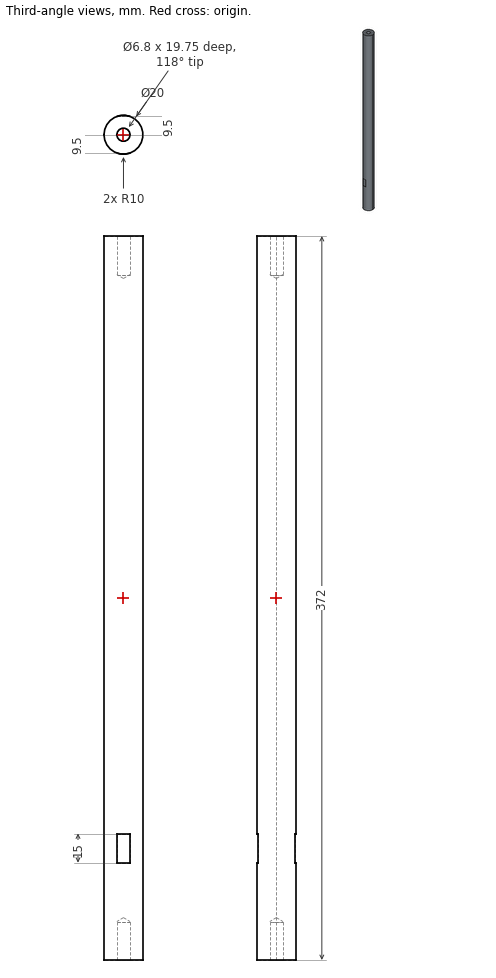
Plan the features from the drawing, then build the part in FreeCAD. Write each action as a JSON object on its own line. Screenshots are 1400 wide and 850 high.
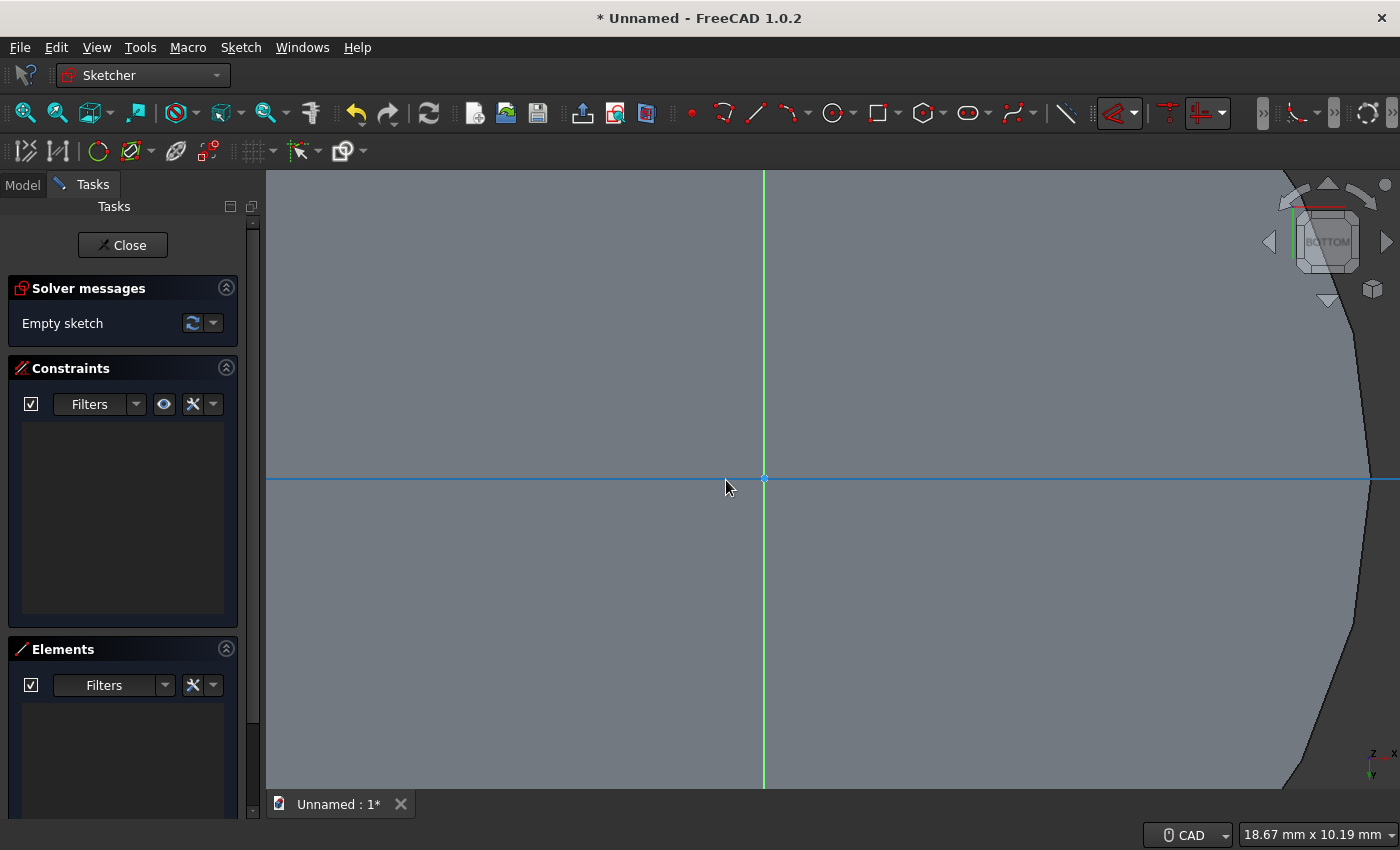
{"action": "left_click", "coordinate": [834, 114]}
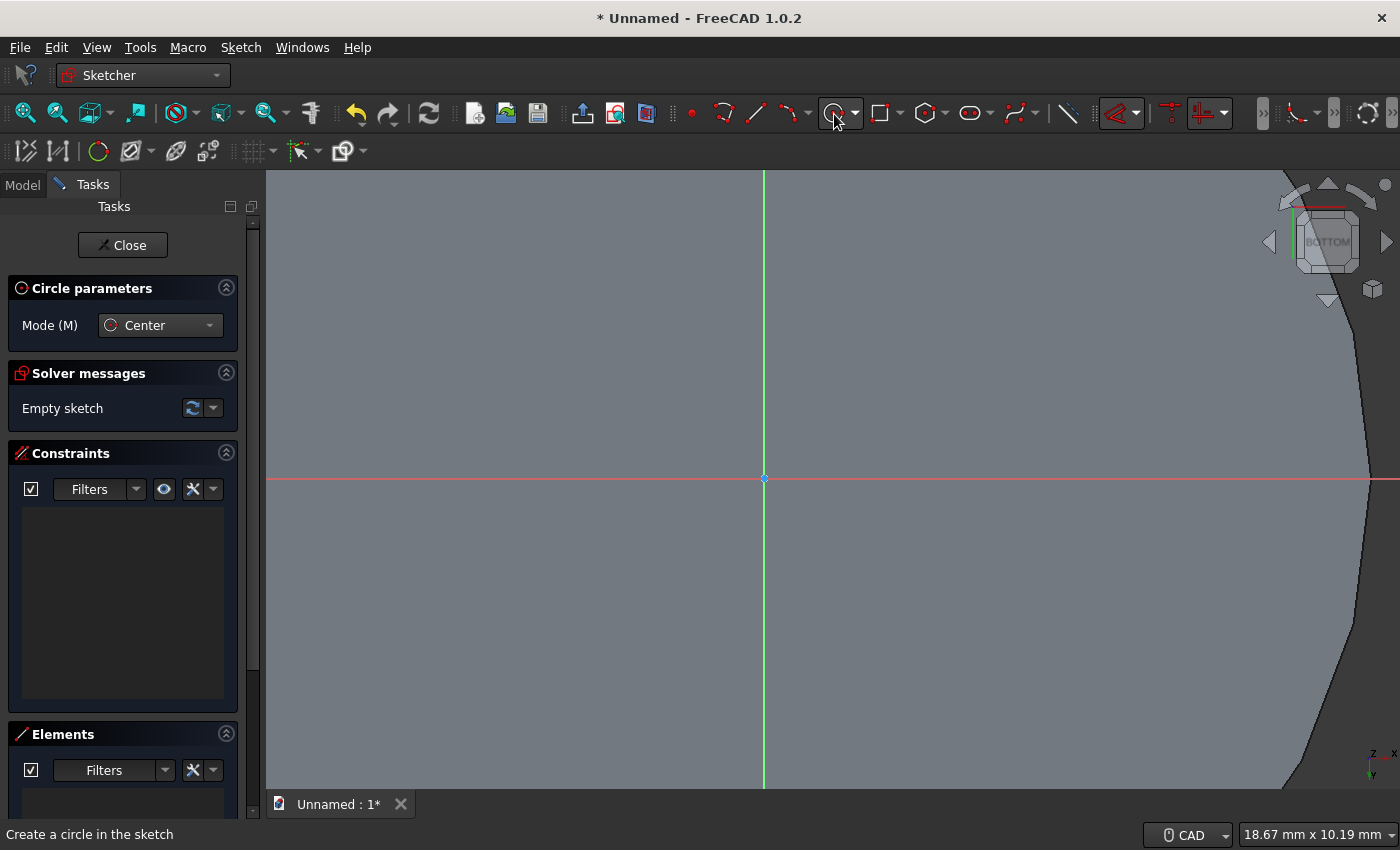
{"action": "left_click", "coordinate": [764, 479]}
{"action": "left_click", "coordinate": [910, 333]}
{"action": "key", "text": "Escape"}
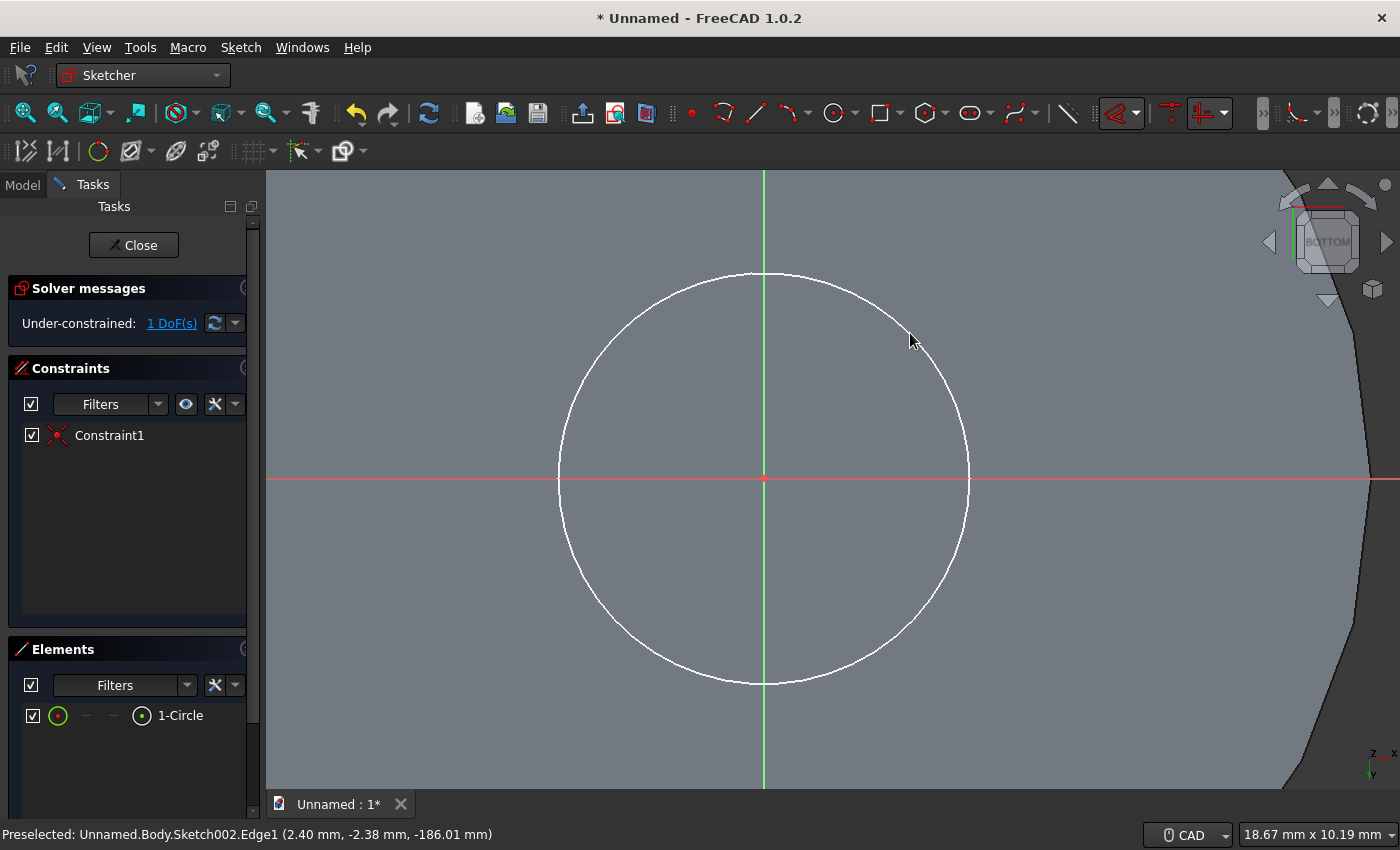
{"action": "left_click", "coordinate": [909, 333]}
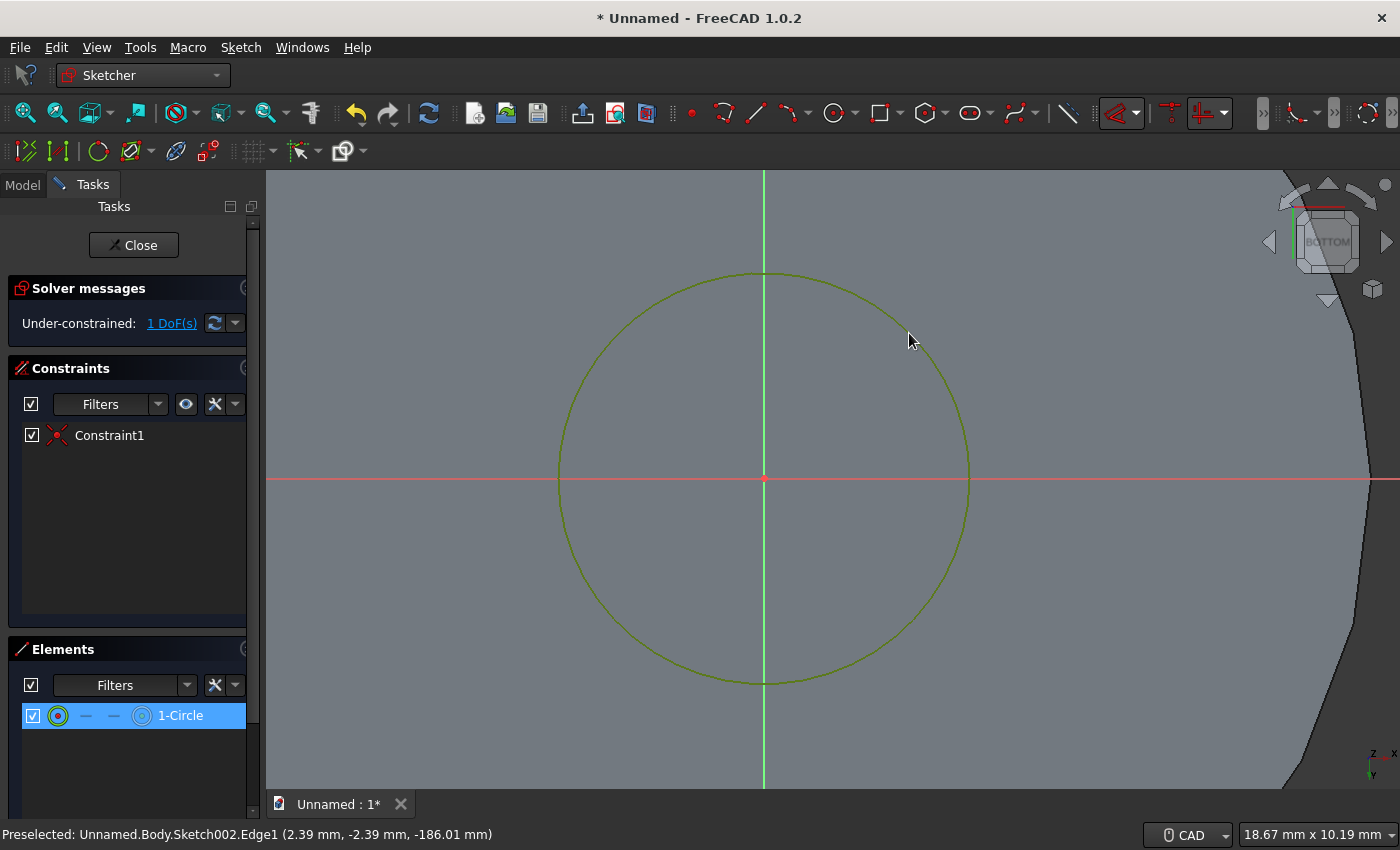
{"action": "left_click", "coordinate": [1138, 114]}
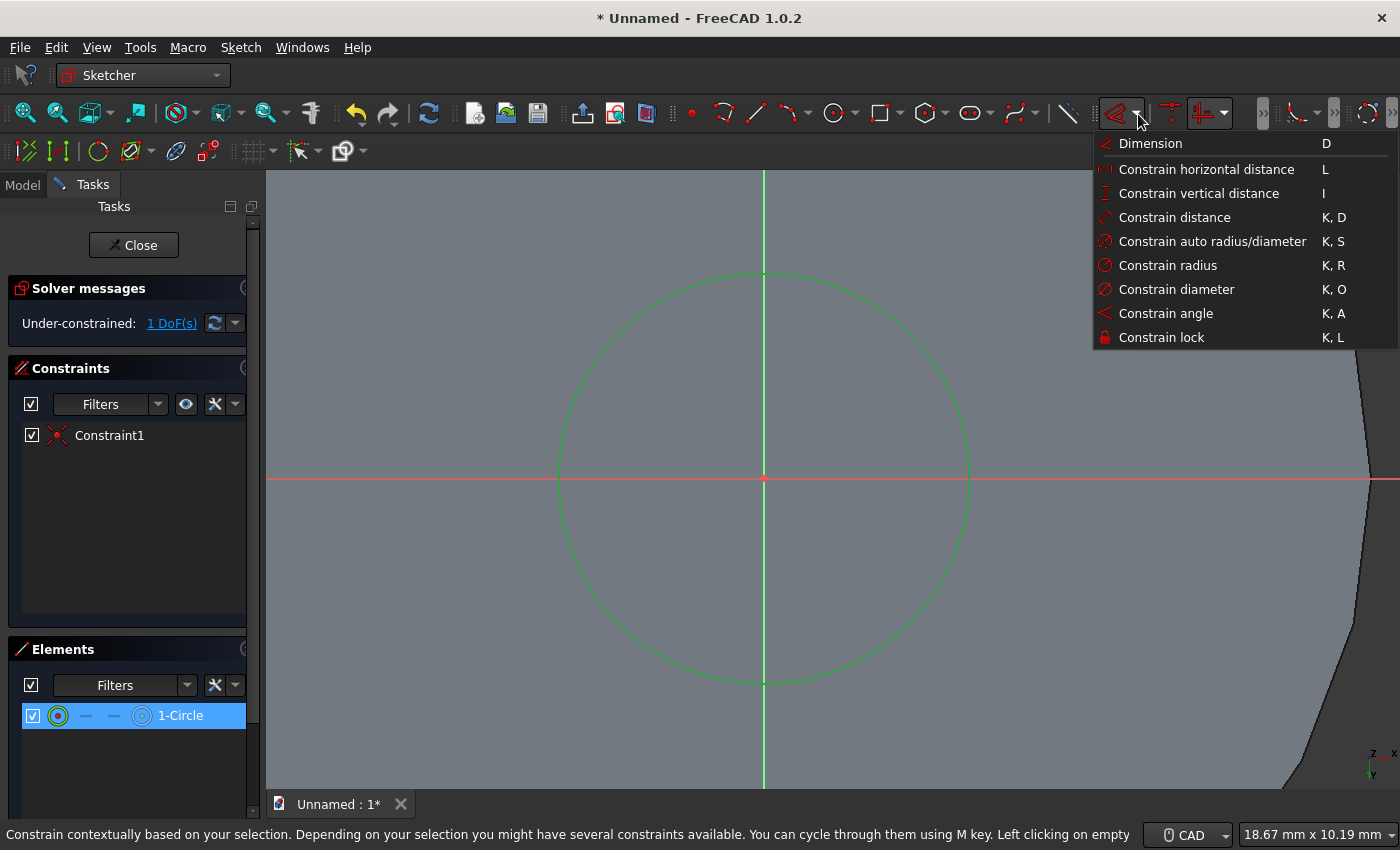
{"action": "left_click", "coordinate": [1246, 289]}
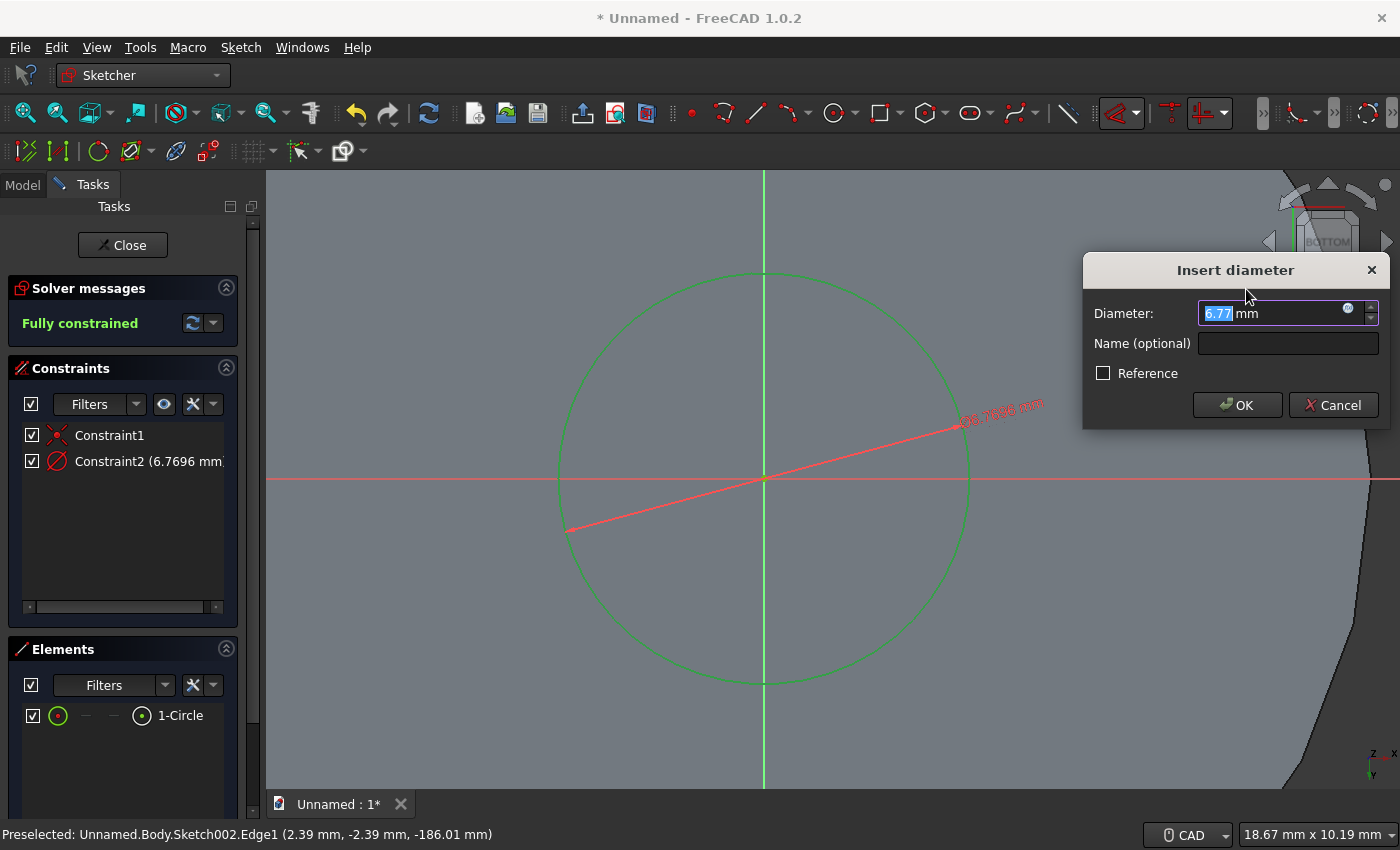
{"action": "type", "text": "6.8"}
{"action": "key", "text": "Return"}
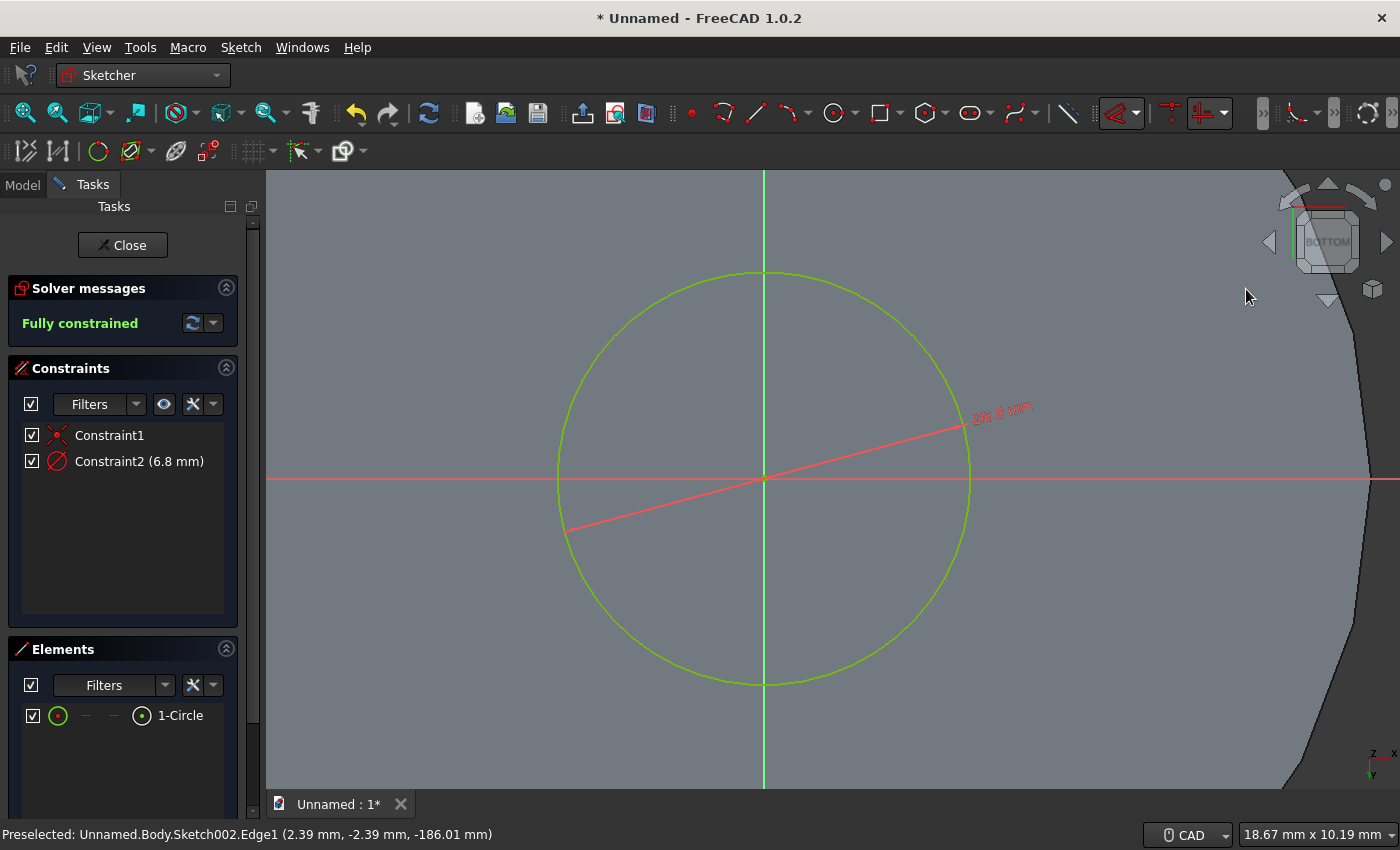
{"action": "left_click", "coordinate": [123, 245]}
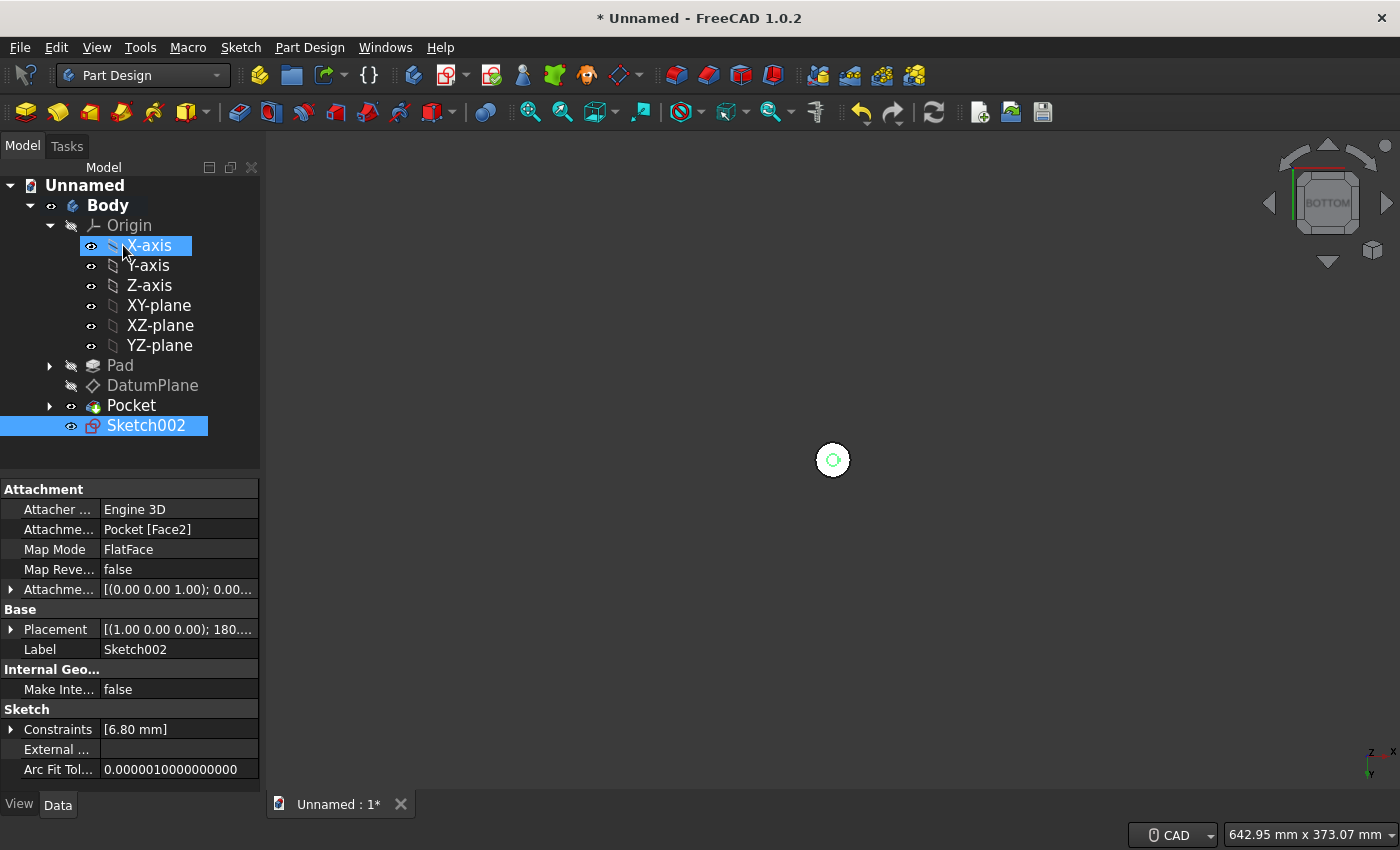
{"action": "left_click", "coordinate": [272, 112]}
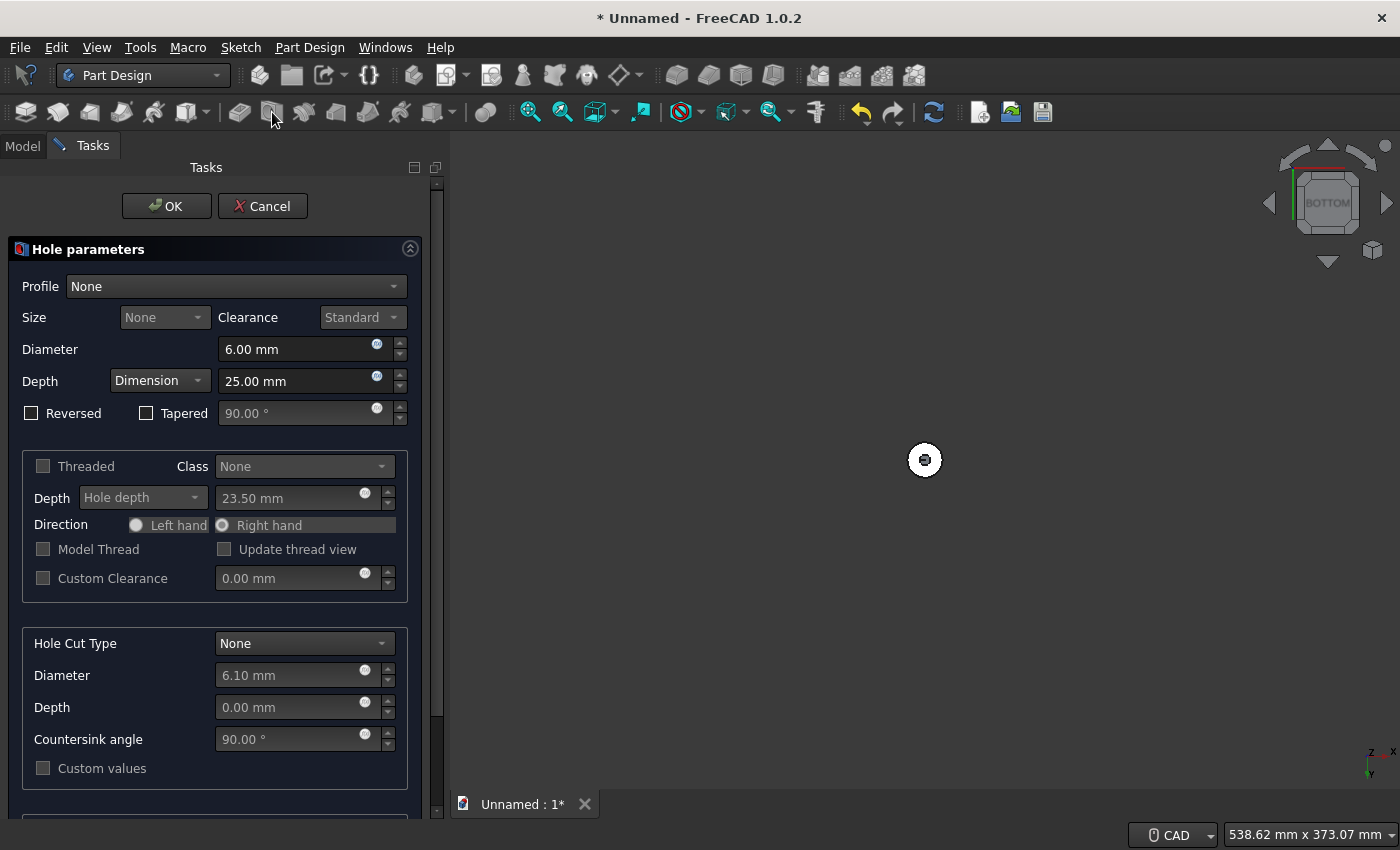
{"action": "triple_click", "coordinate": [305, 349]}